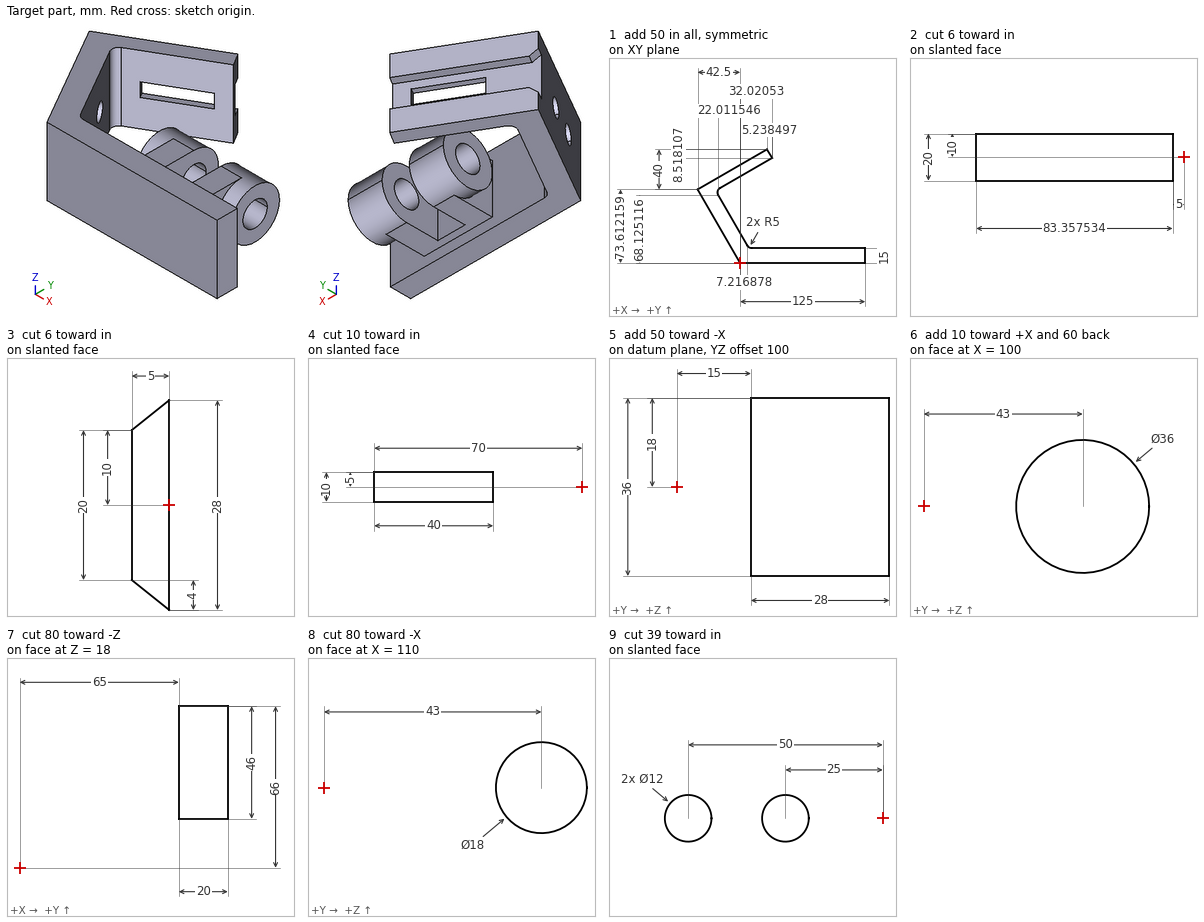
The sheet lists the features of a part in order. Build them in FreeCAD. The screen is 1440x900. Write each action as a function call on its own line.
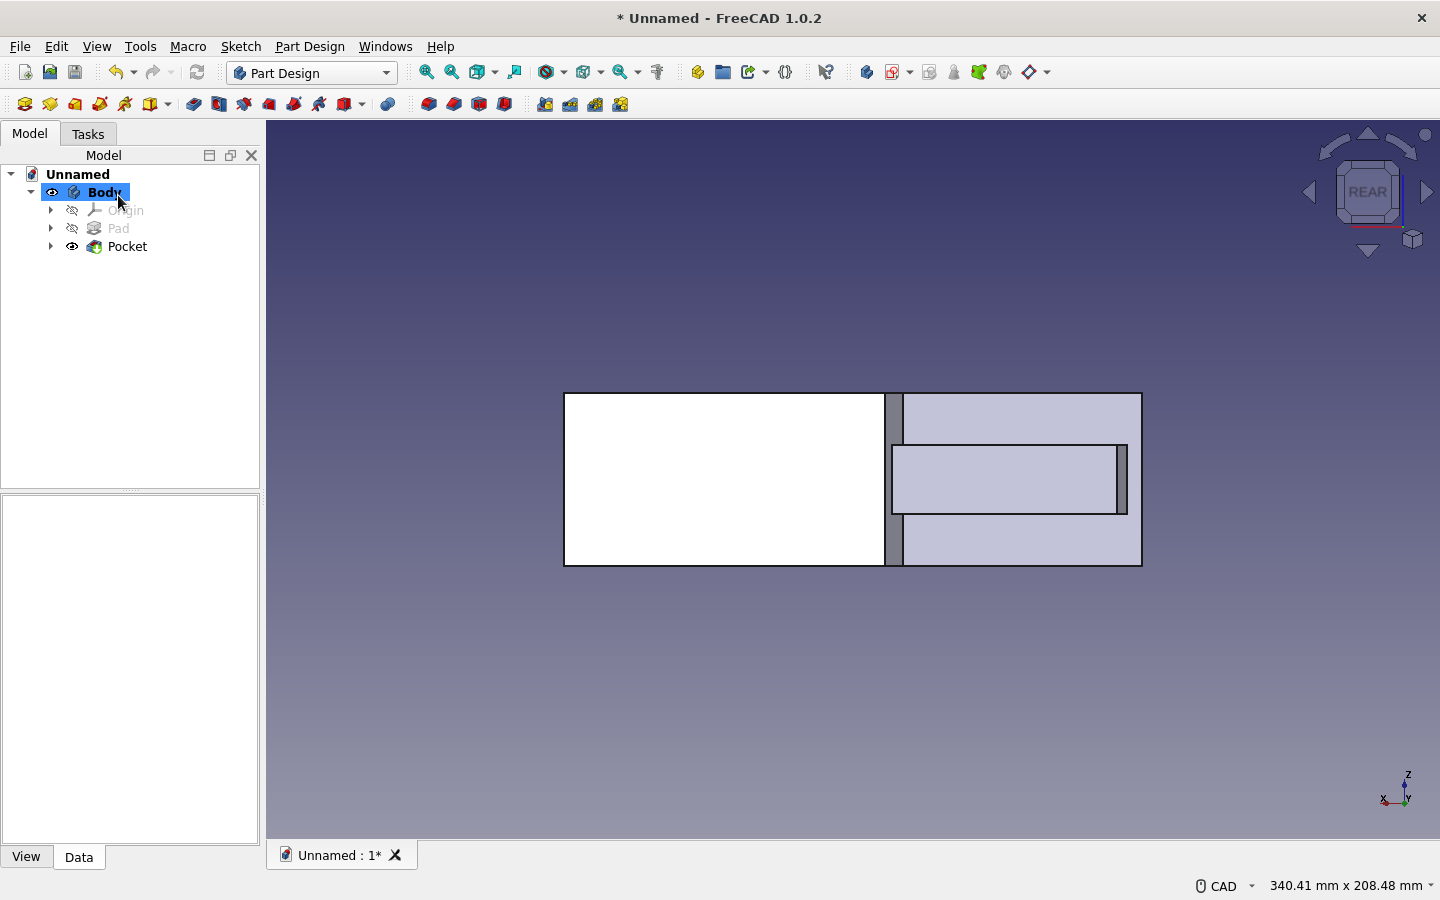
click(920, 528)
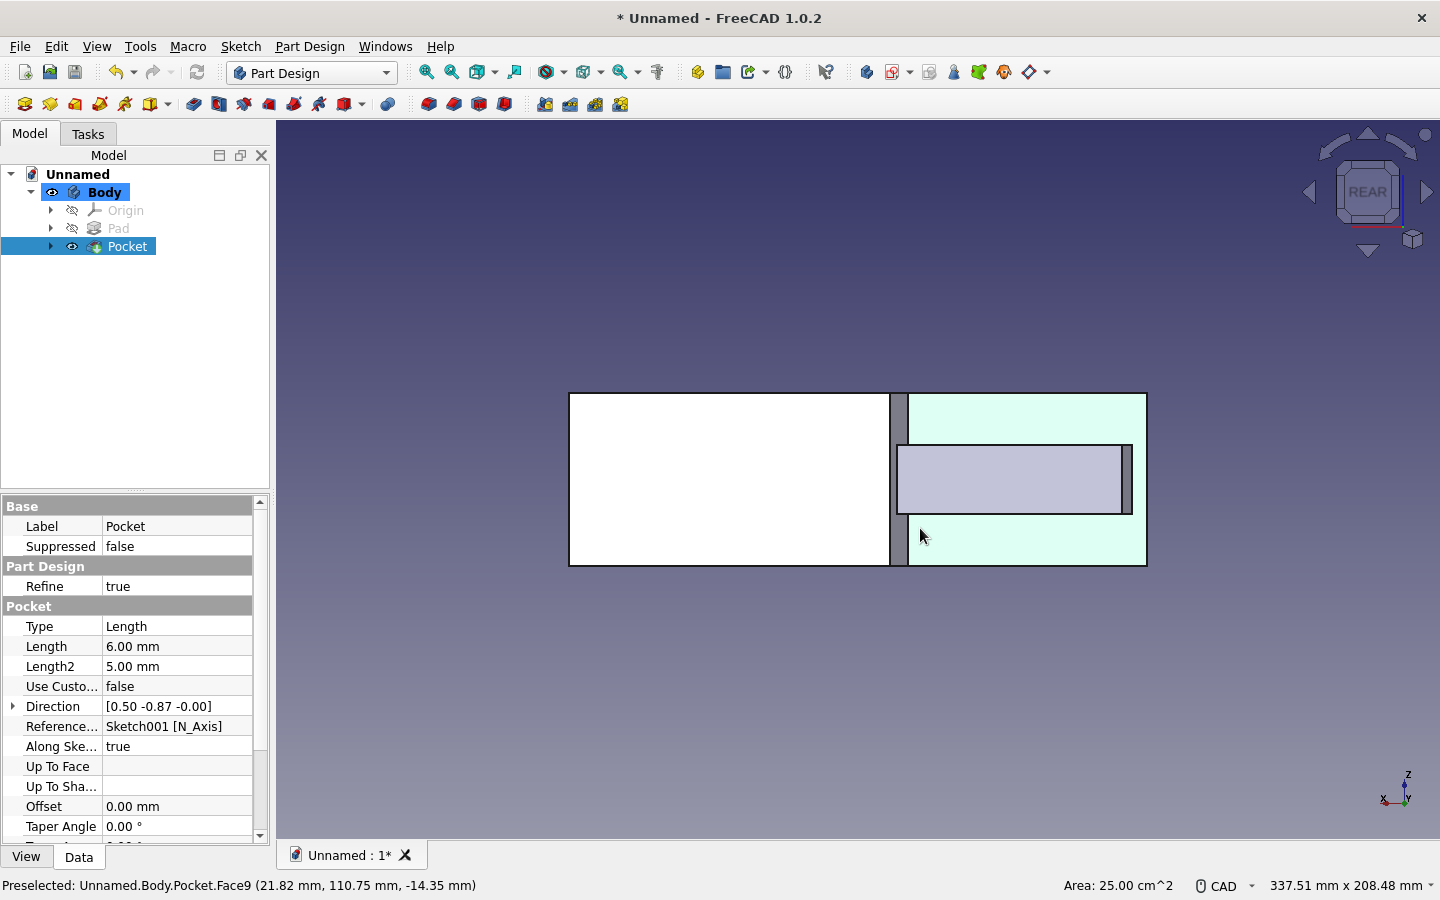
click(892, 72)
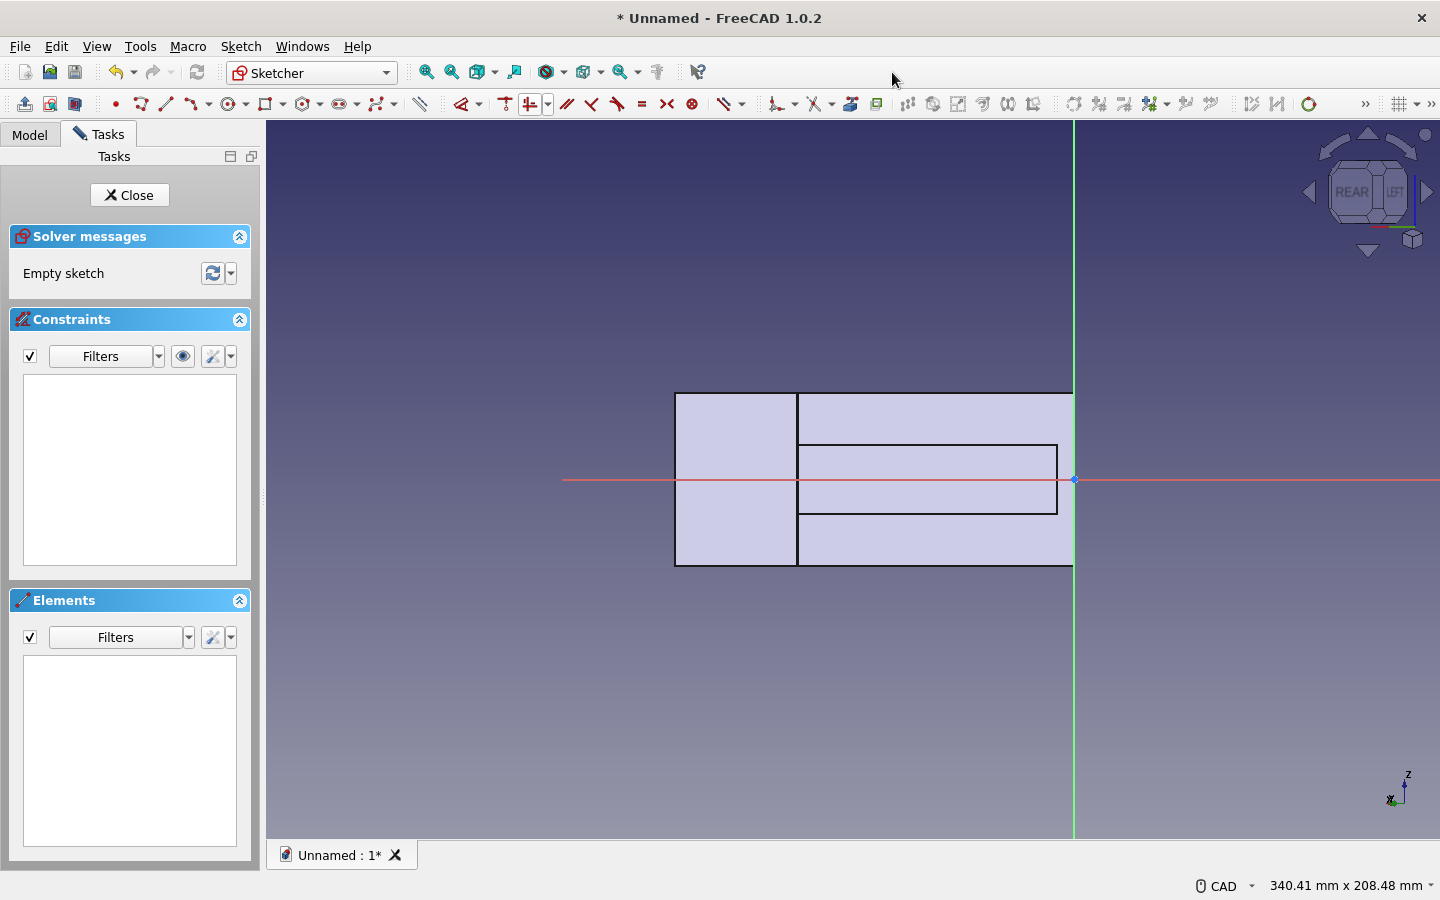
scroll(1137, 480, up, 8)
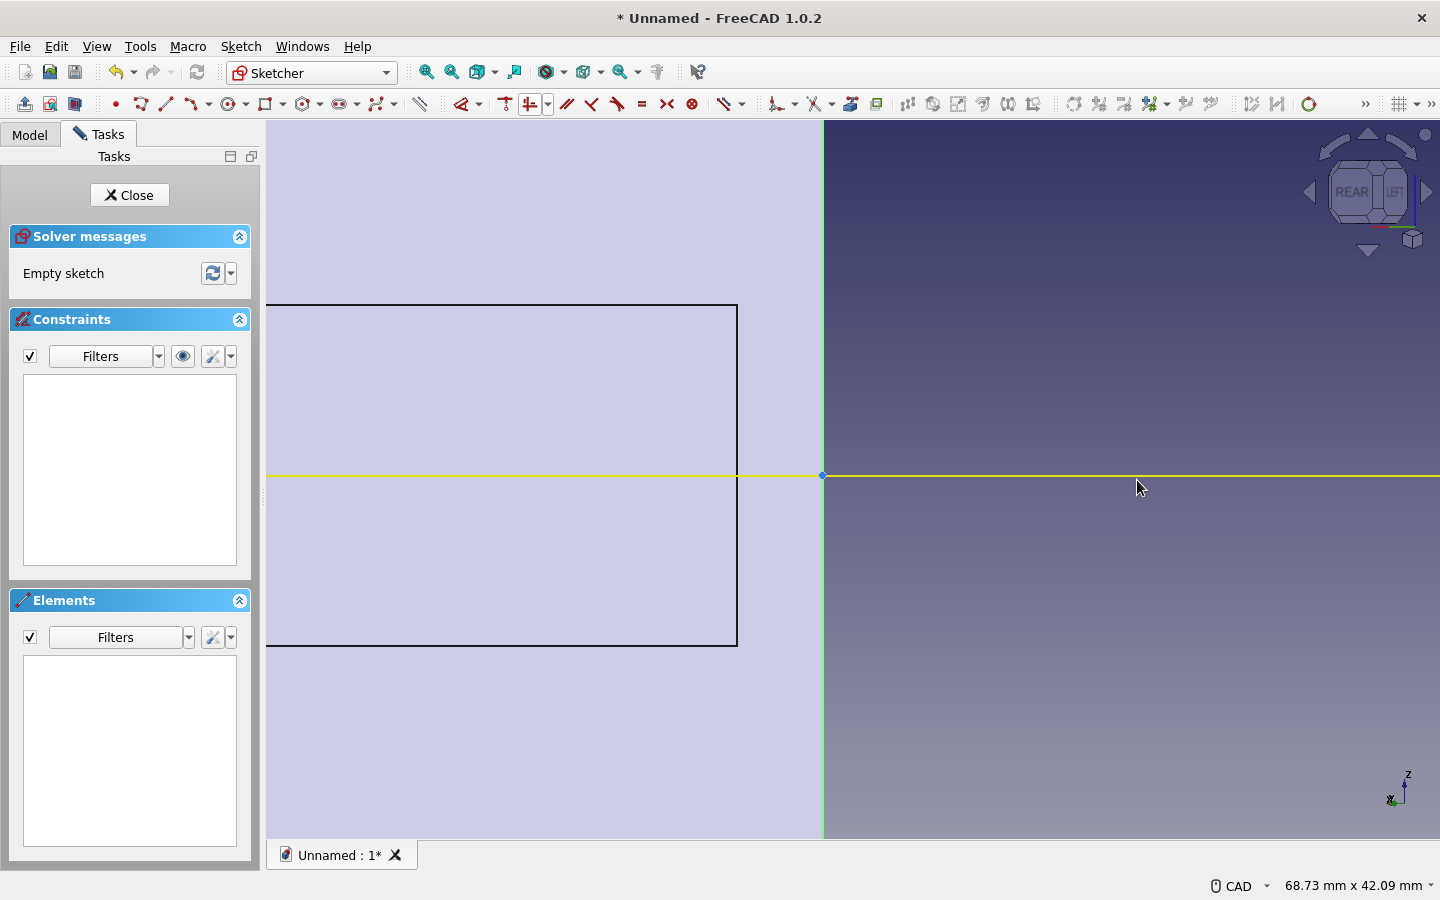
key(g)
key(m)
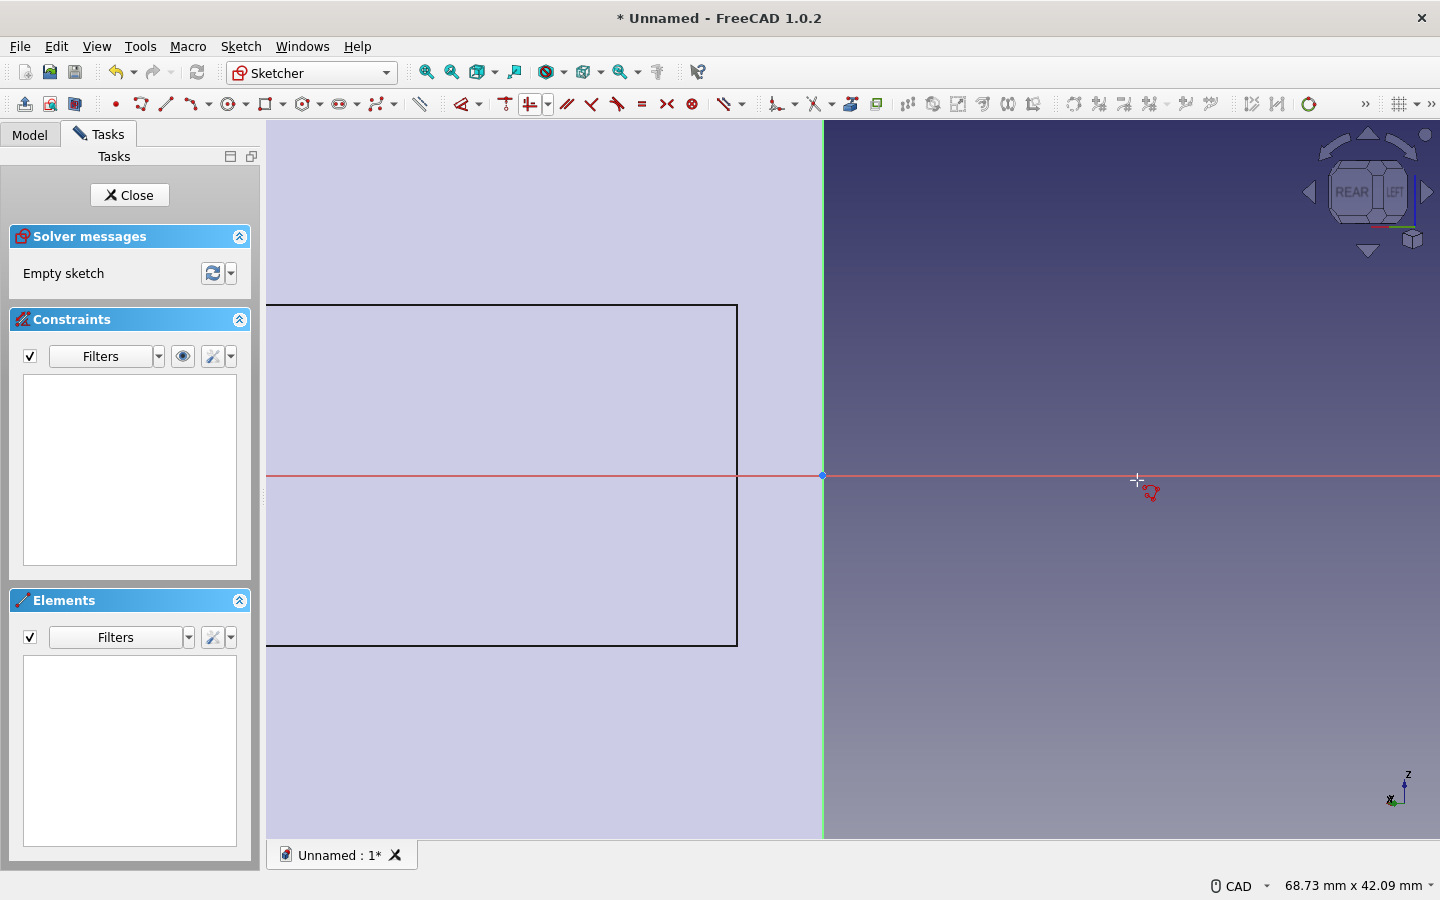
click(737, 305)
click(737, 646)
click(823, 715)
click(814, 236)
click(737, 306)
key(Escape)
key(Escape)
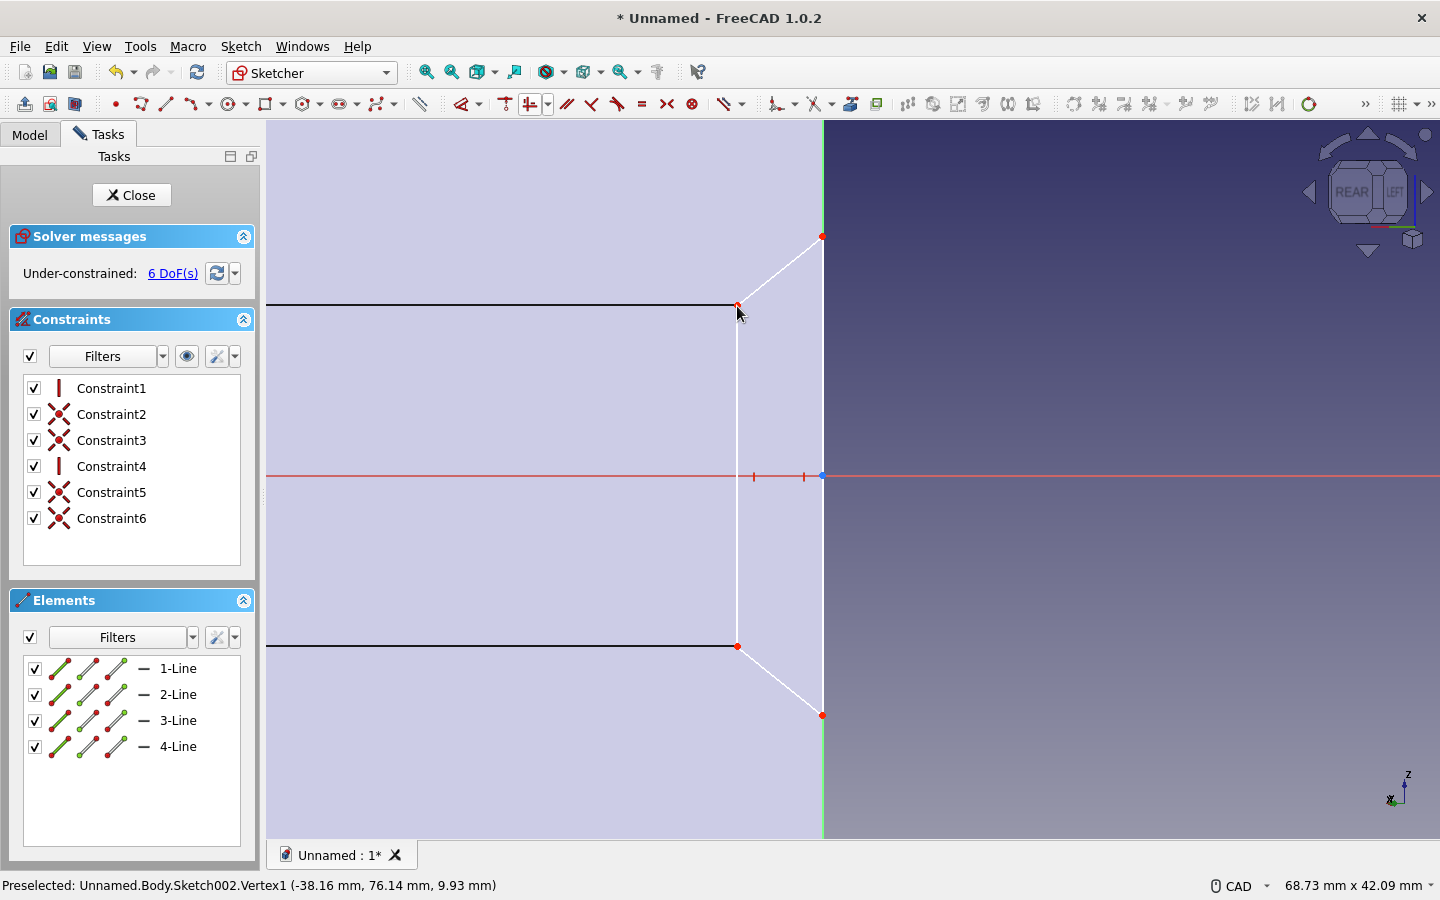
click(823, 716)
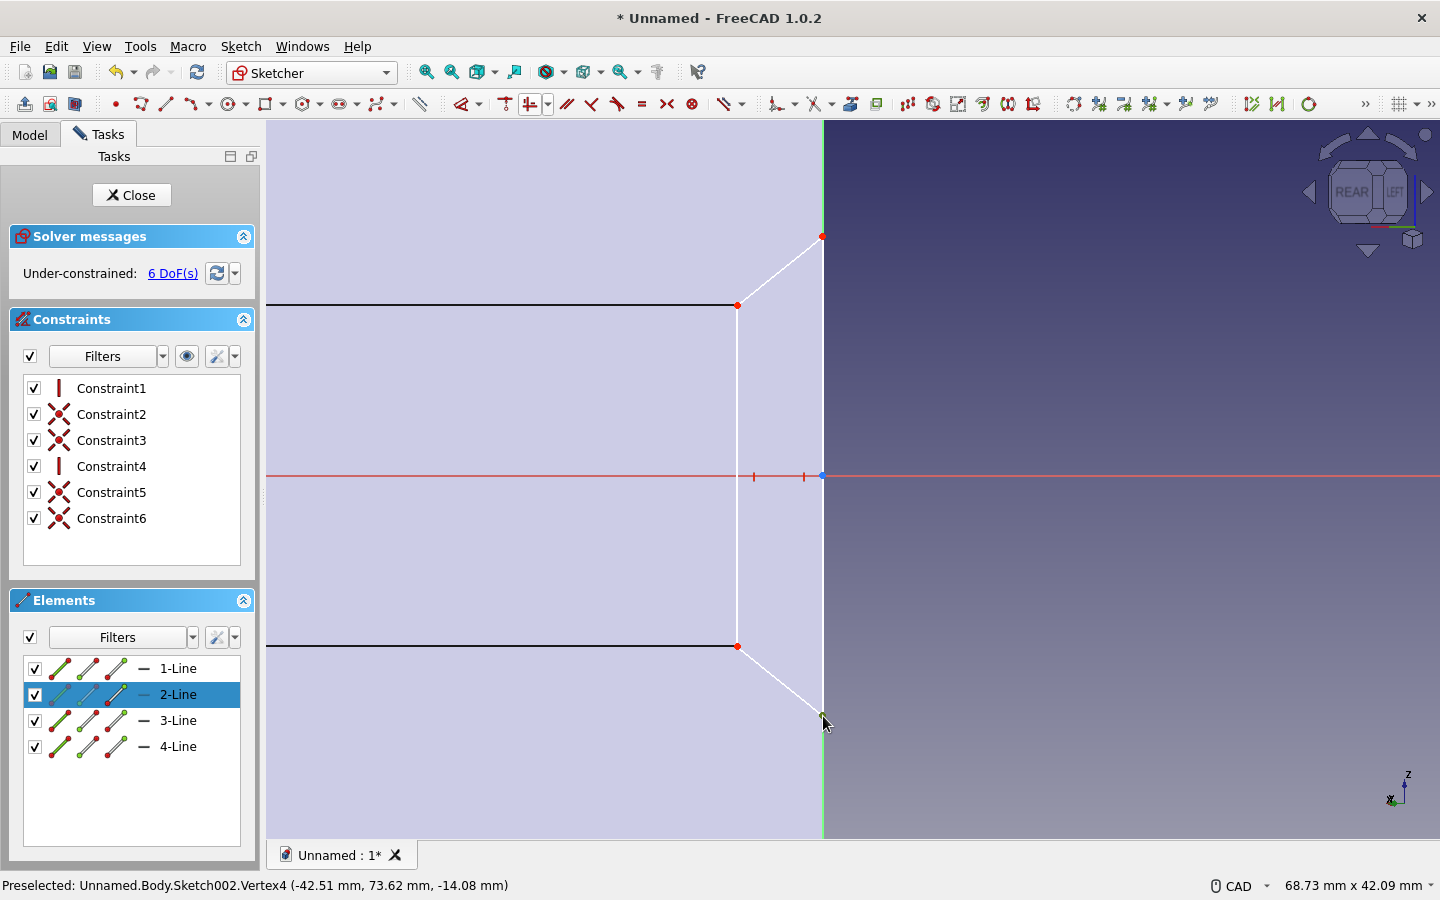
click(823, 764)